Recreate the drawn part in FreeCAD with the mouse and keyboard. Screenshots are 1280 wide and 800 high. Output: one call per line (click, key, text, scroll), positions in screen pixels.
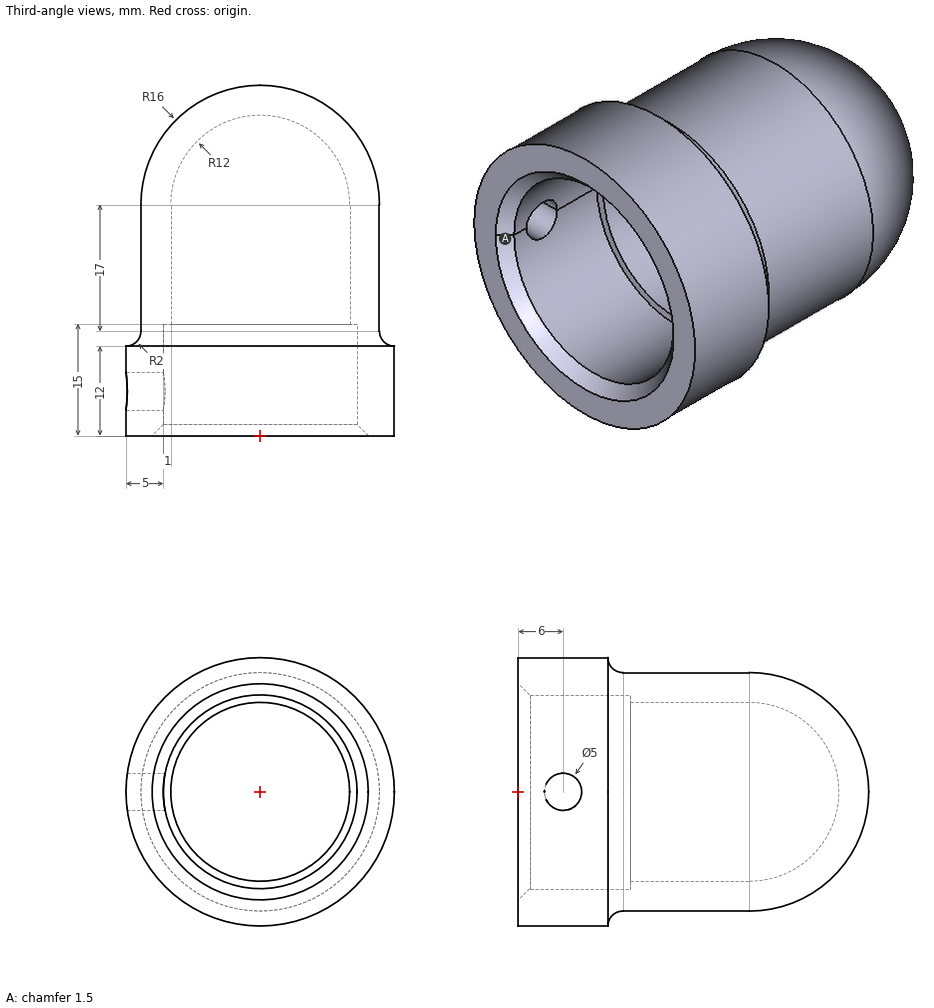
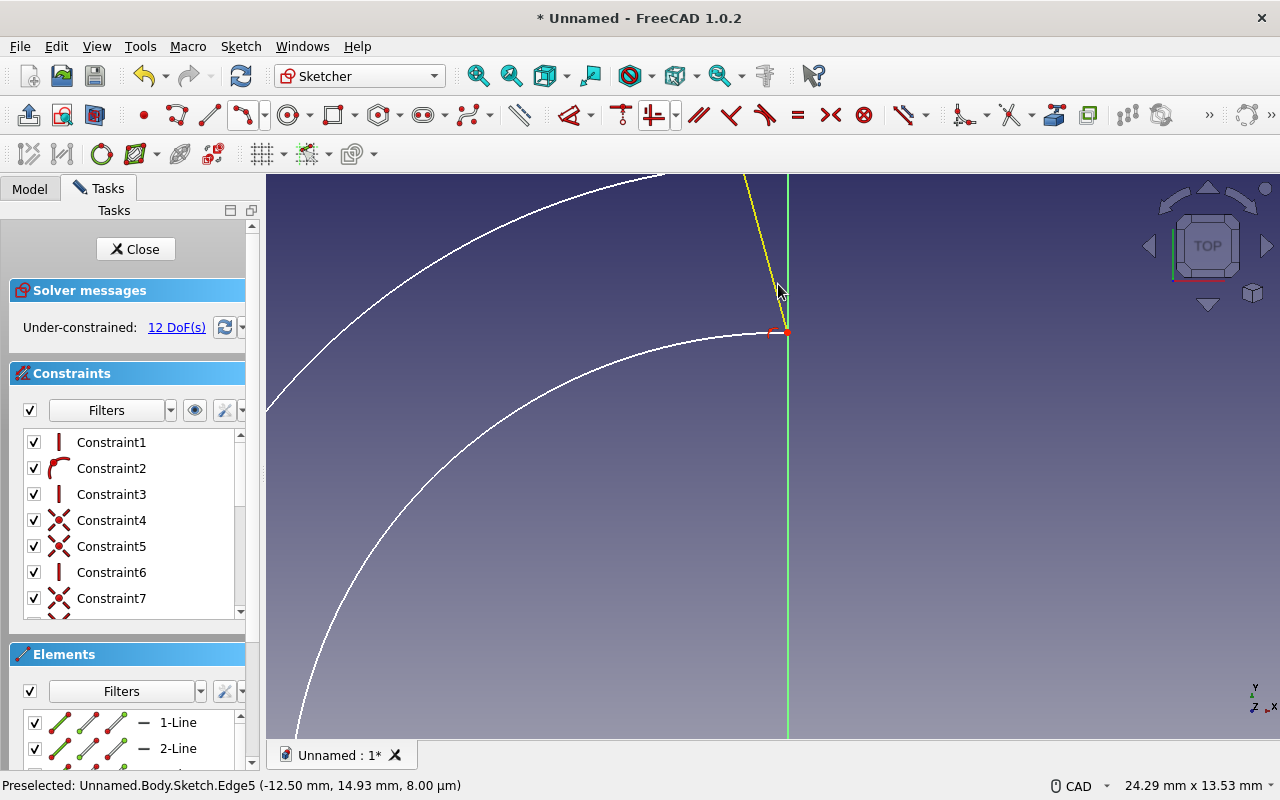
click(774, 282)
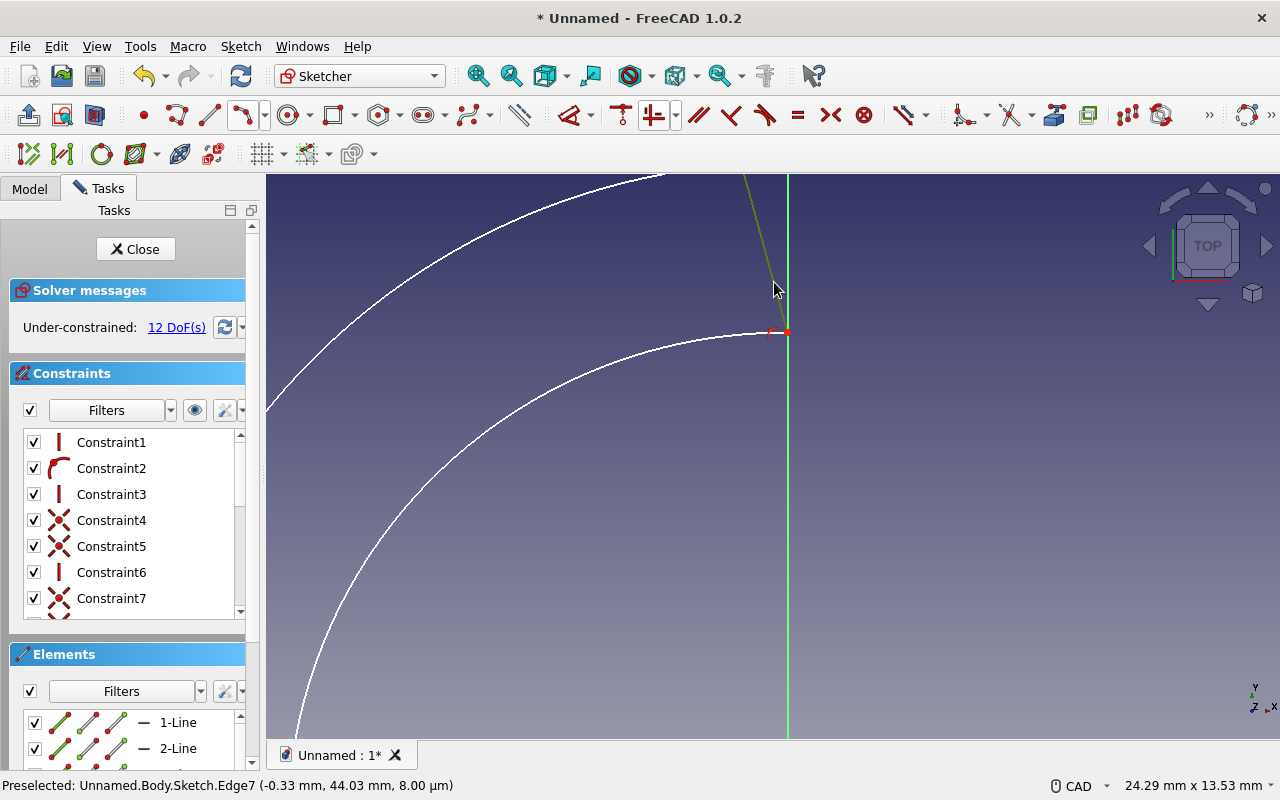
key(v)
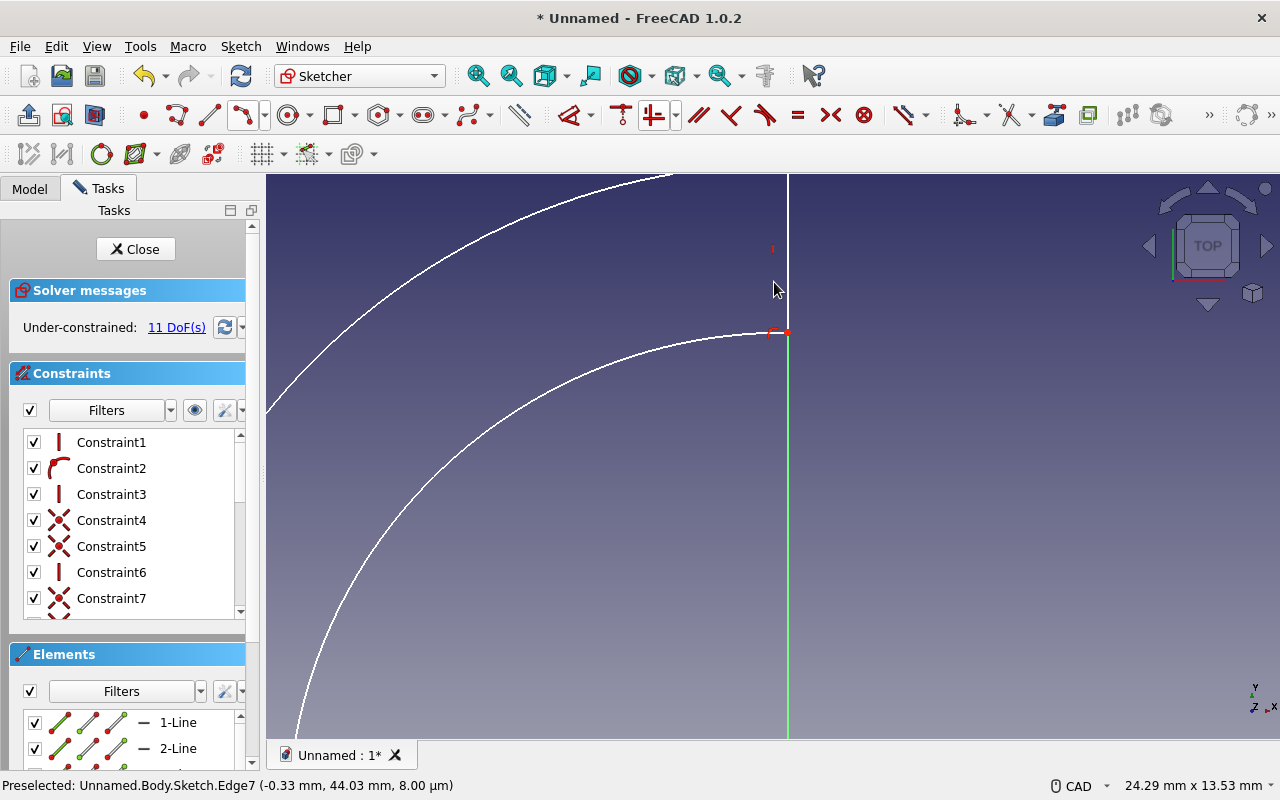
scroll(779, 284, down, 8)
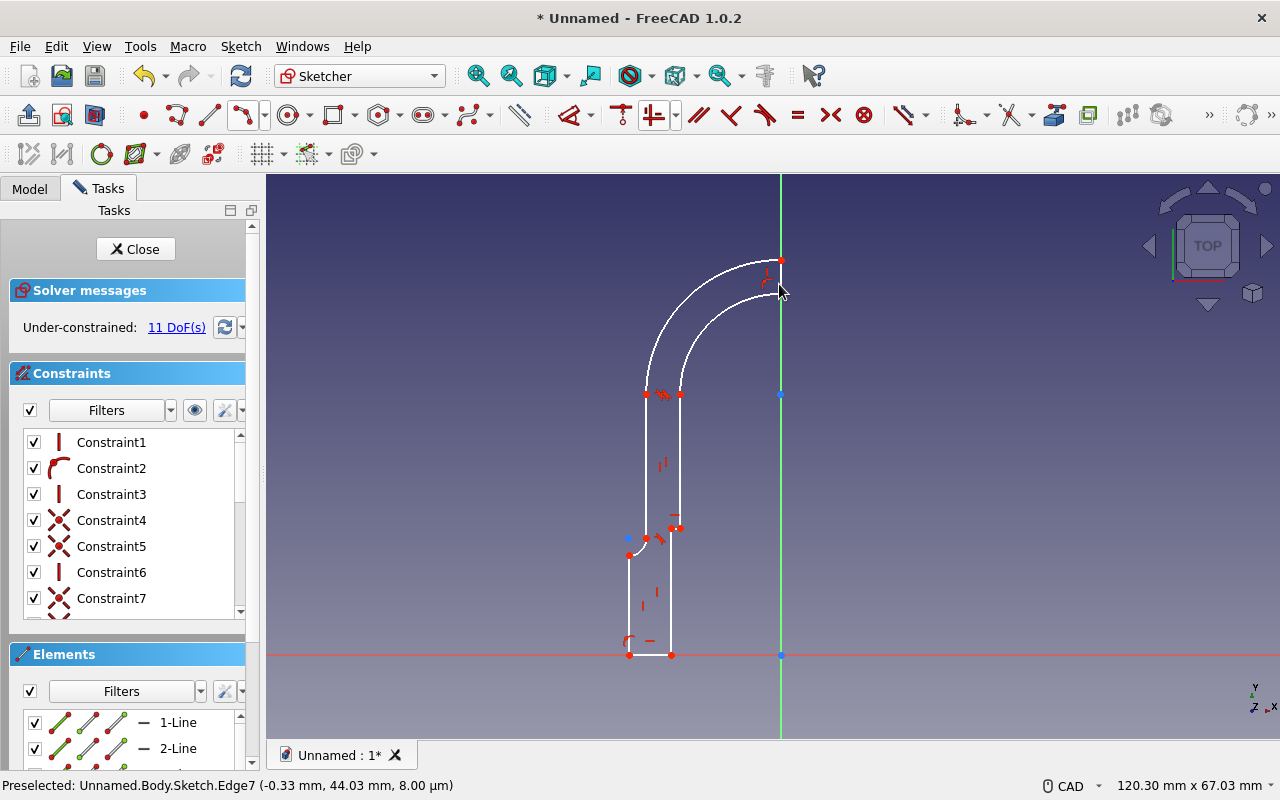
click(735, 305)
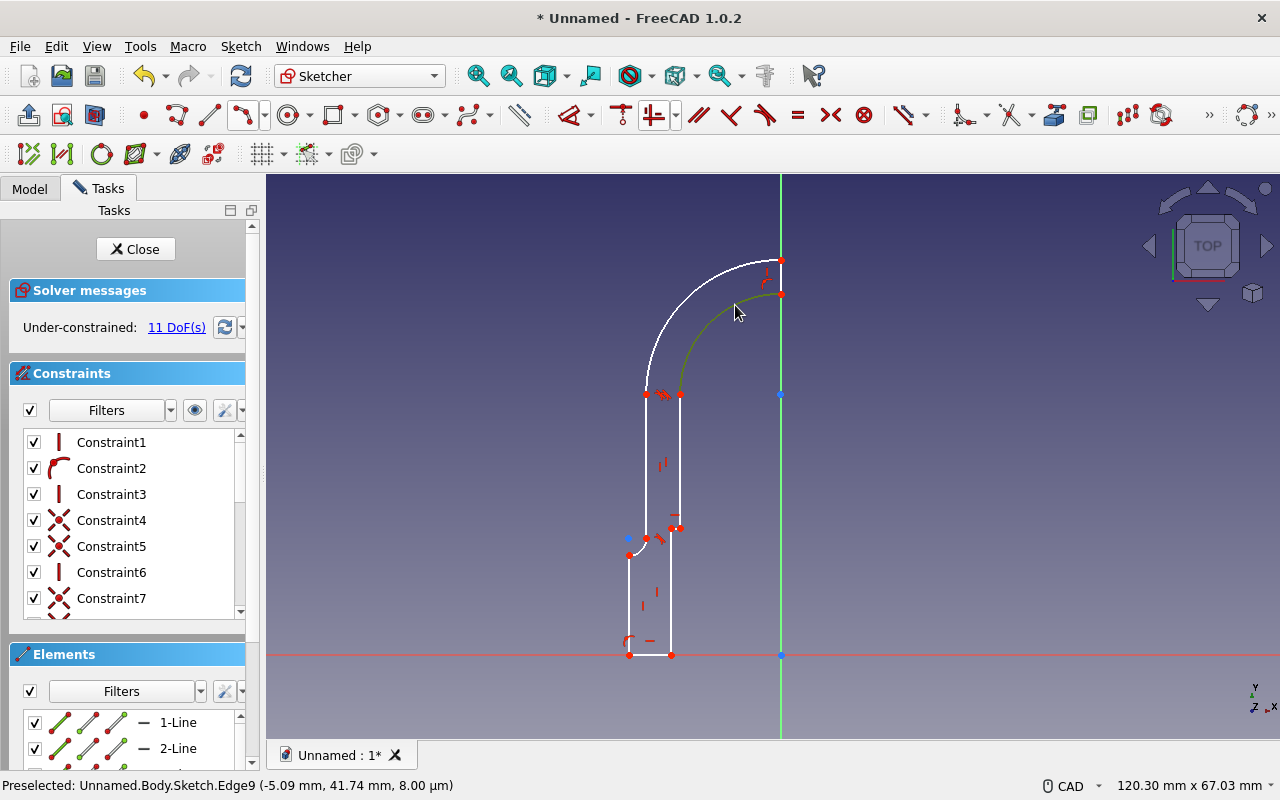
click(720, 275)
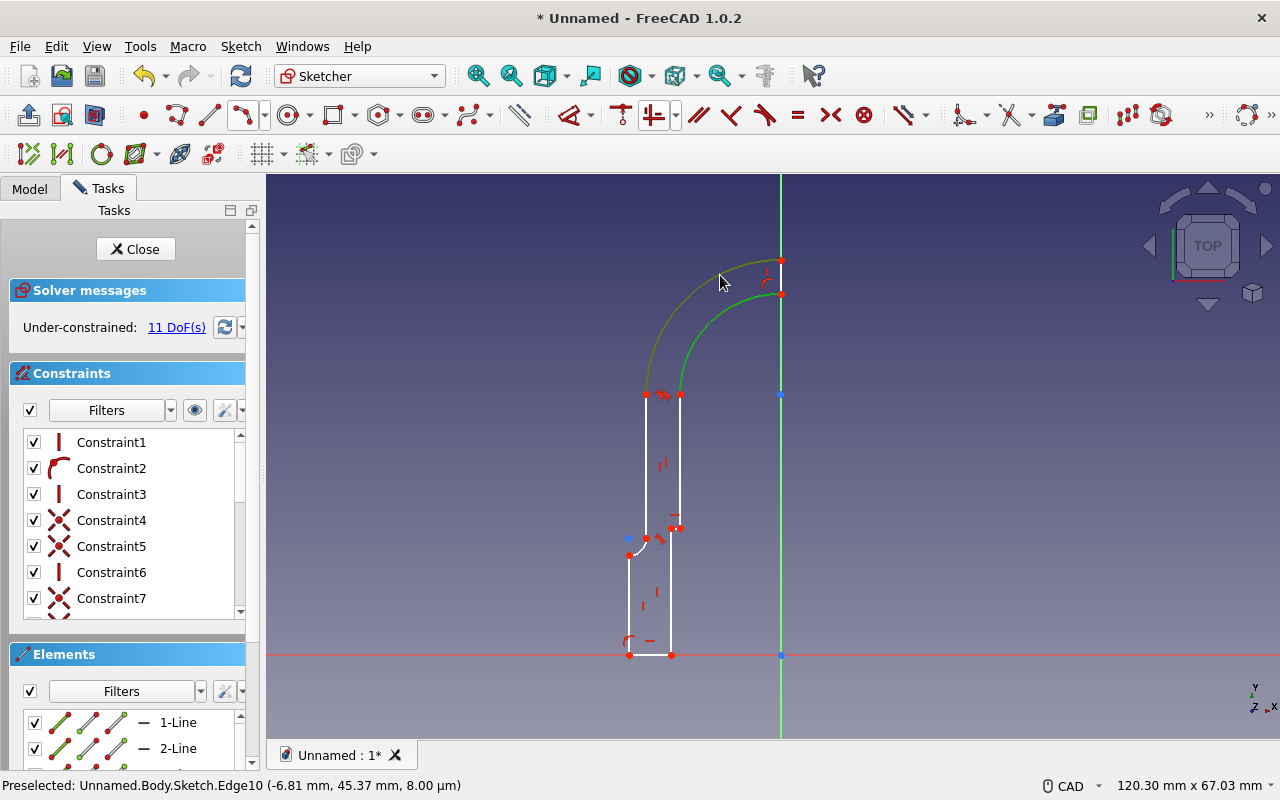
click(621, 116)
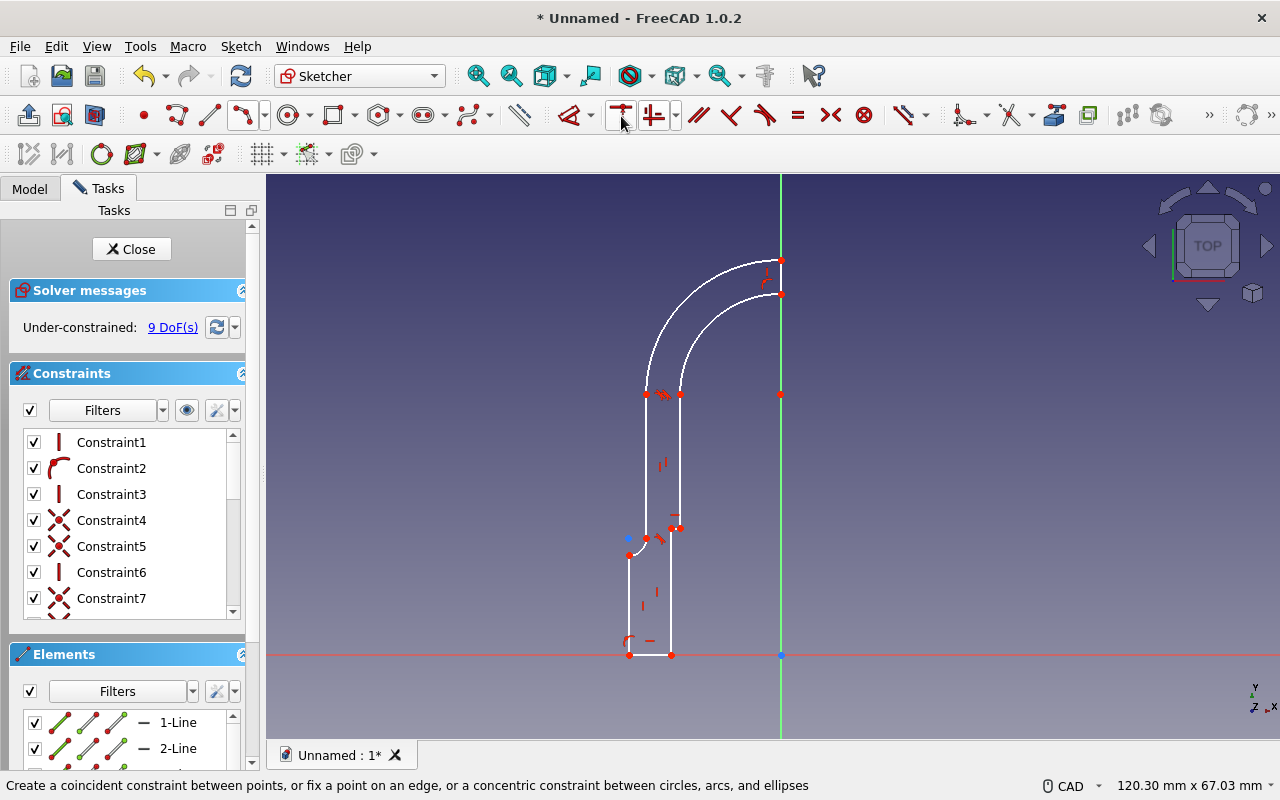
click(781, 395)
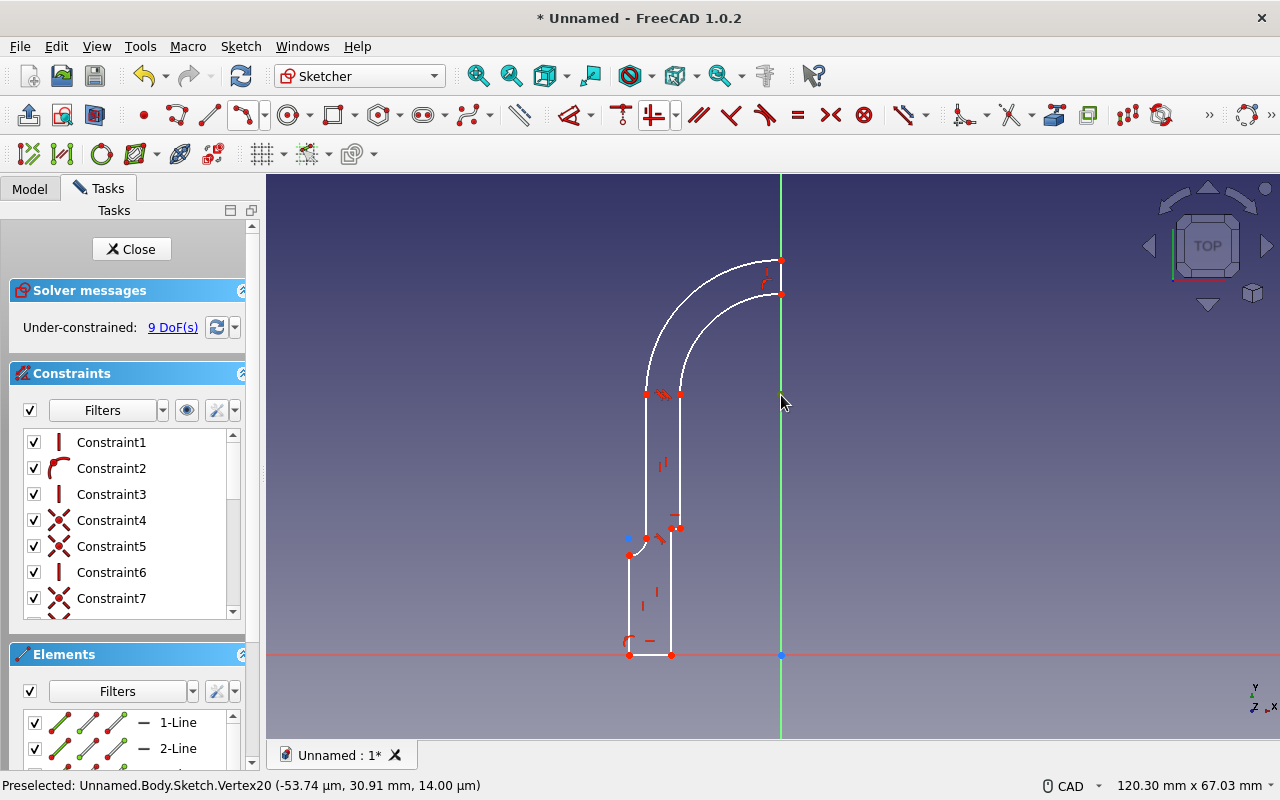
click(781, 602)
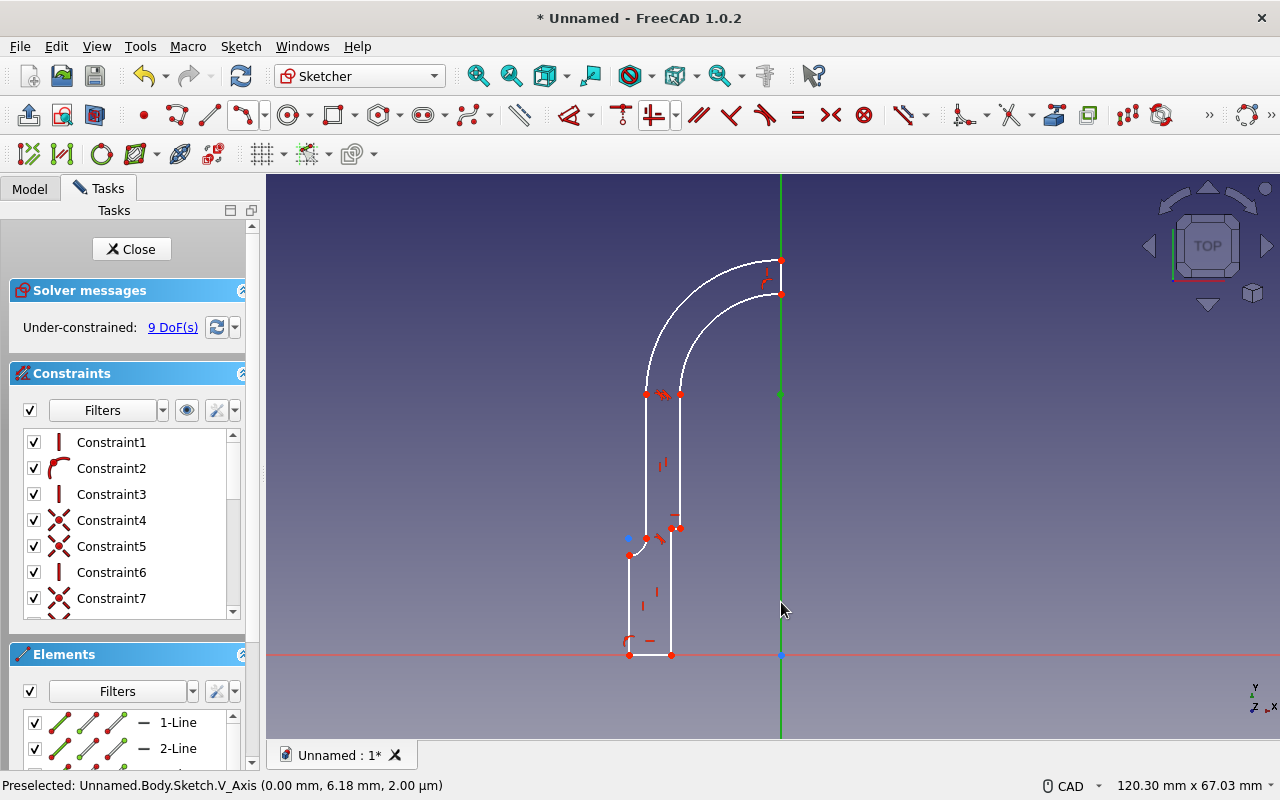
click(621, 116)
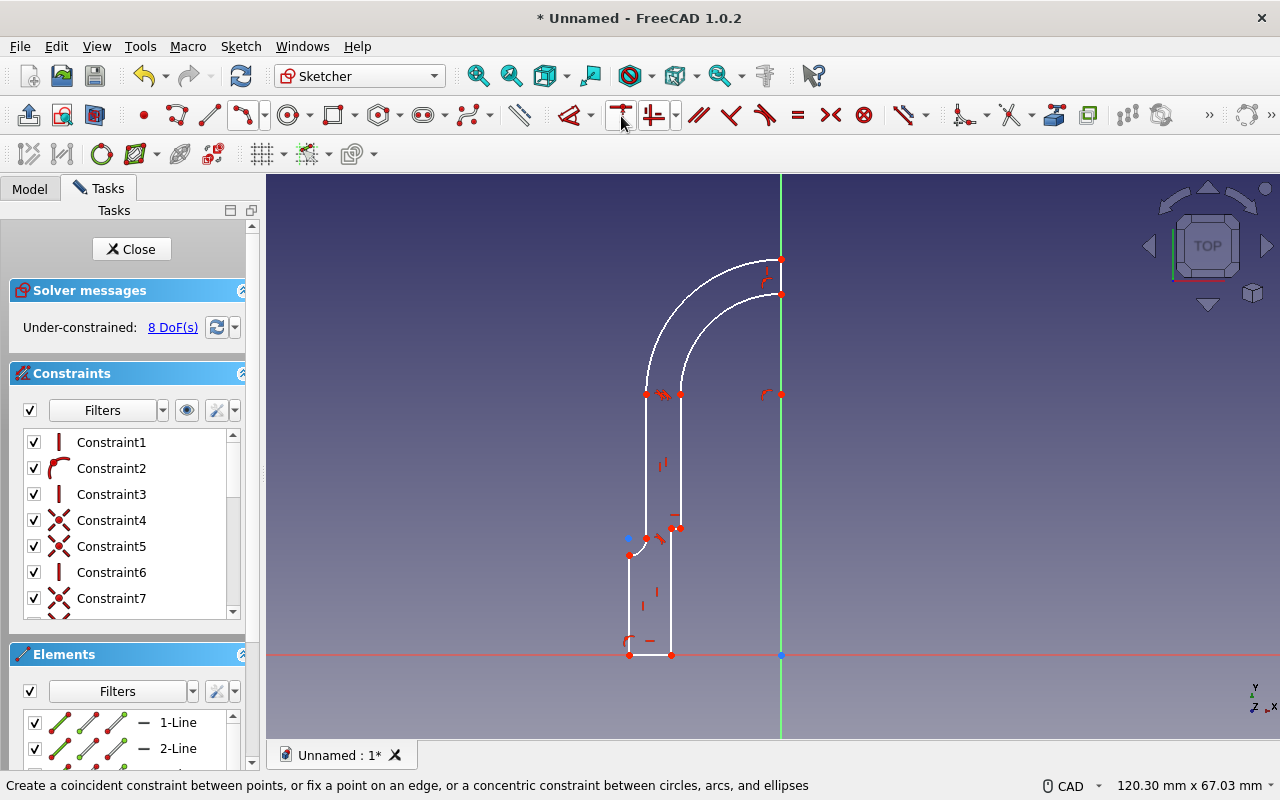
click(568, 116)